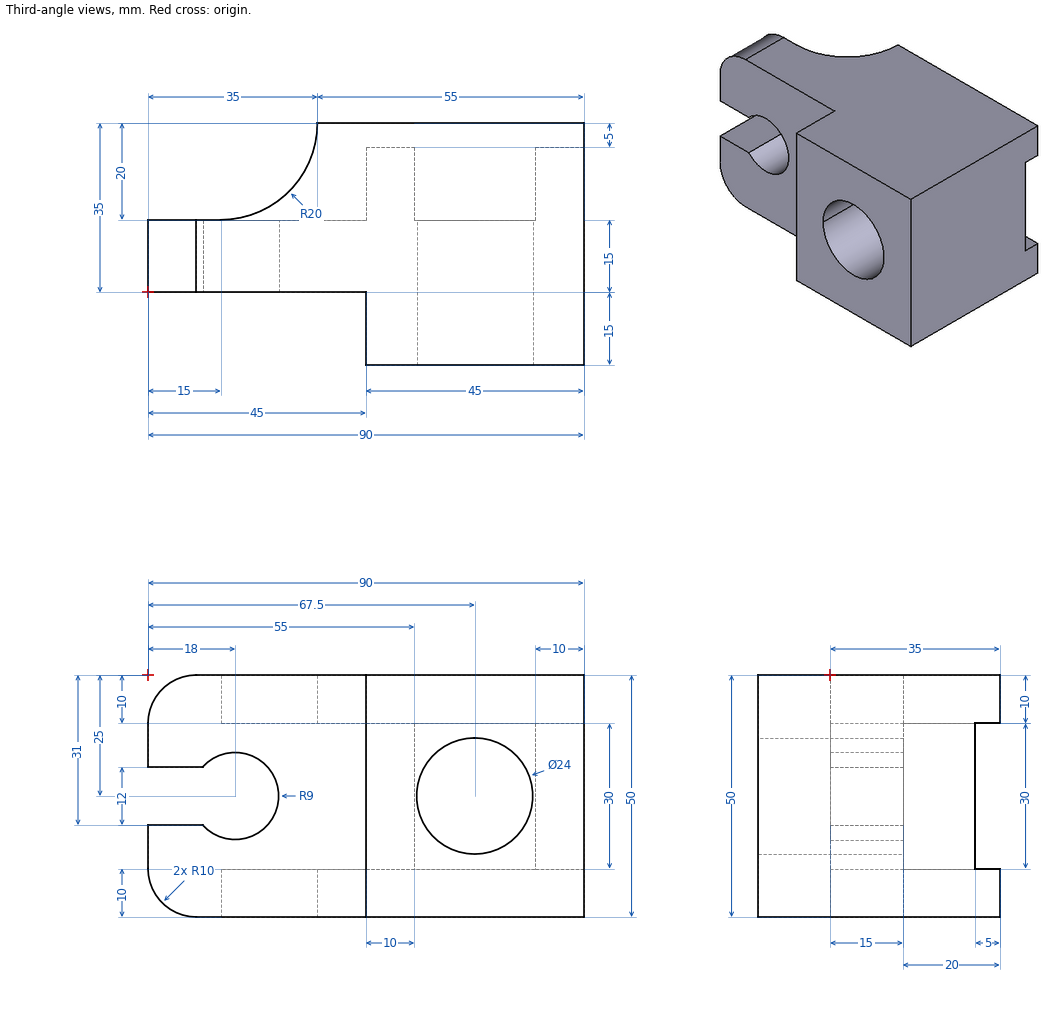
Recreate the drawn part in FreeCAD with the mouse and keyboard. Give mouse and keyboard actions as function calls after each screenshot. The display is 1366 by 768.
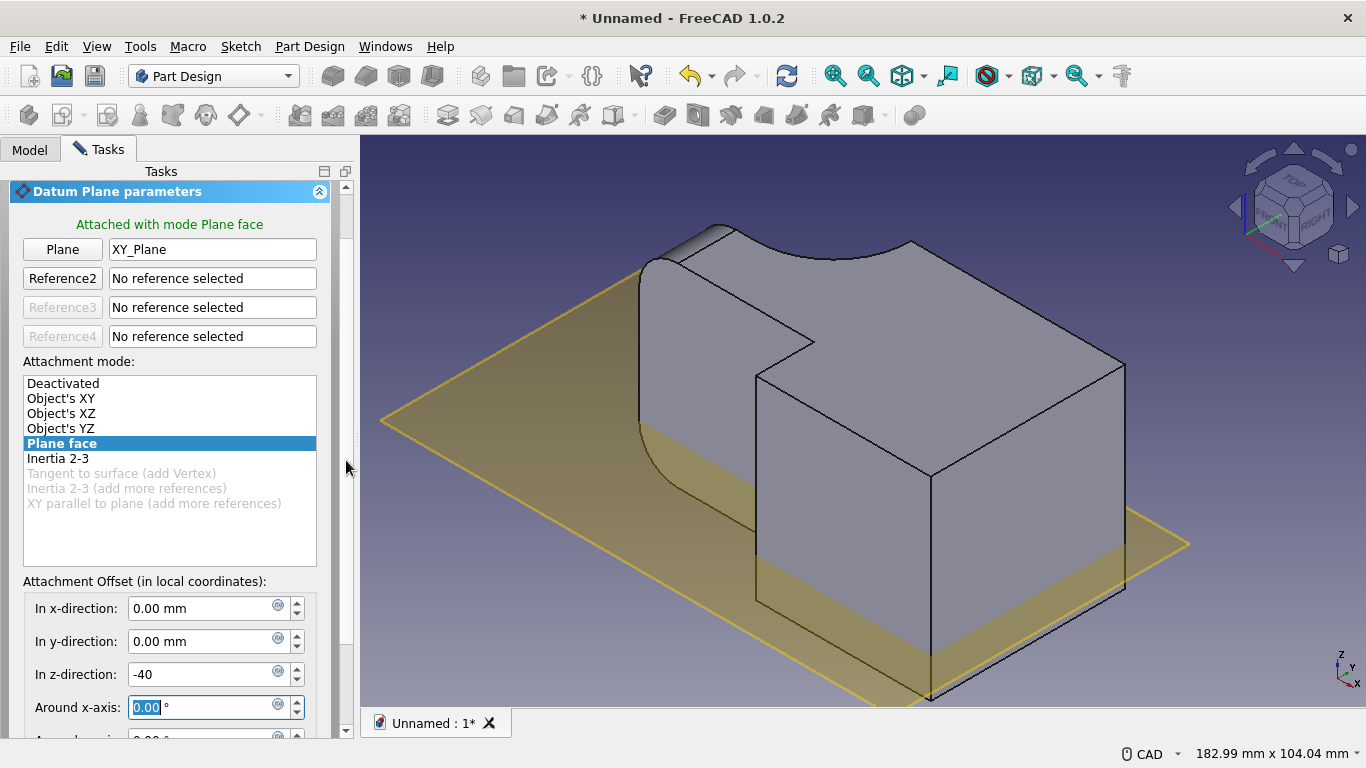
click(127, 210)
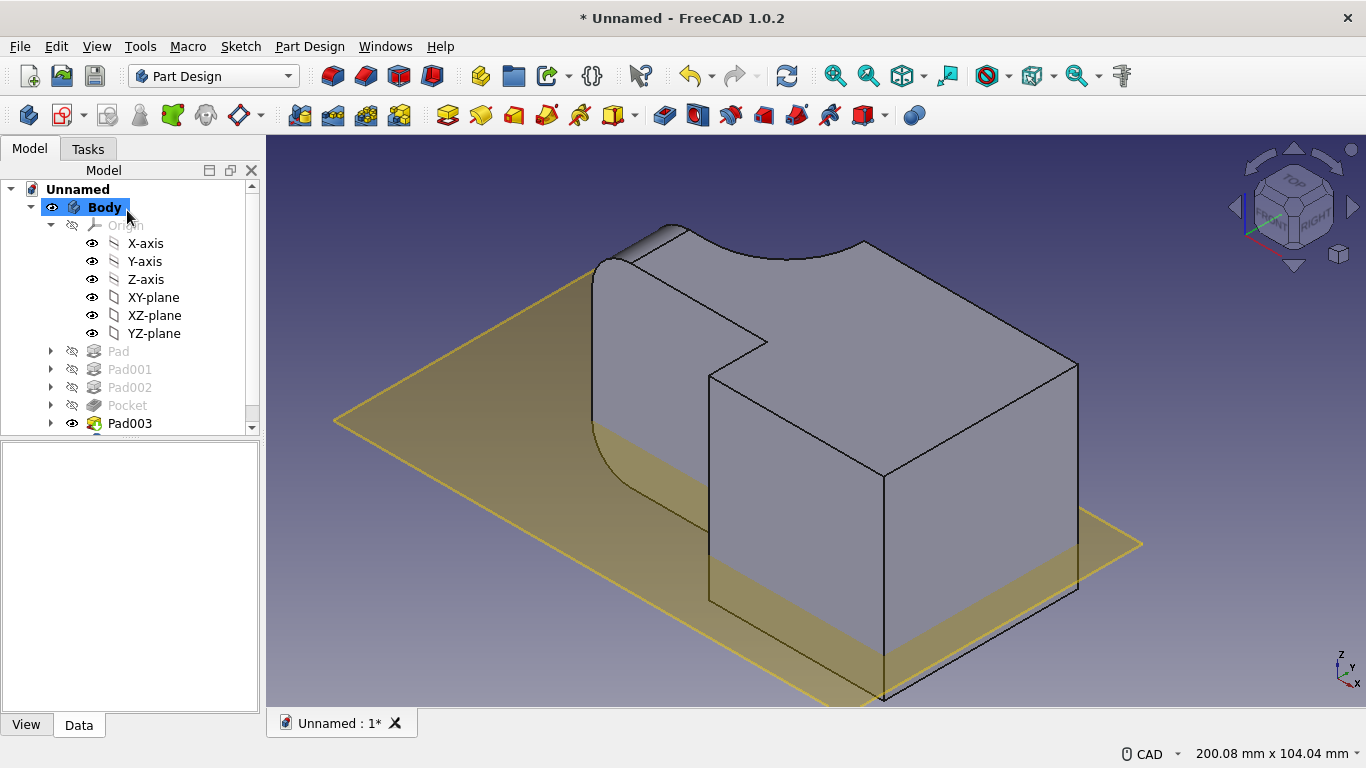
scroll(101, 311, down, 3)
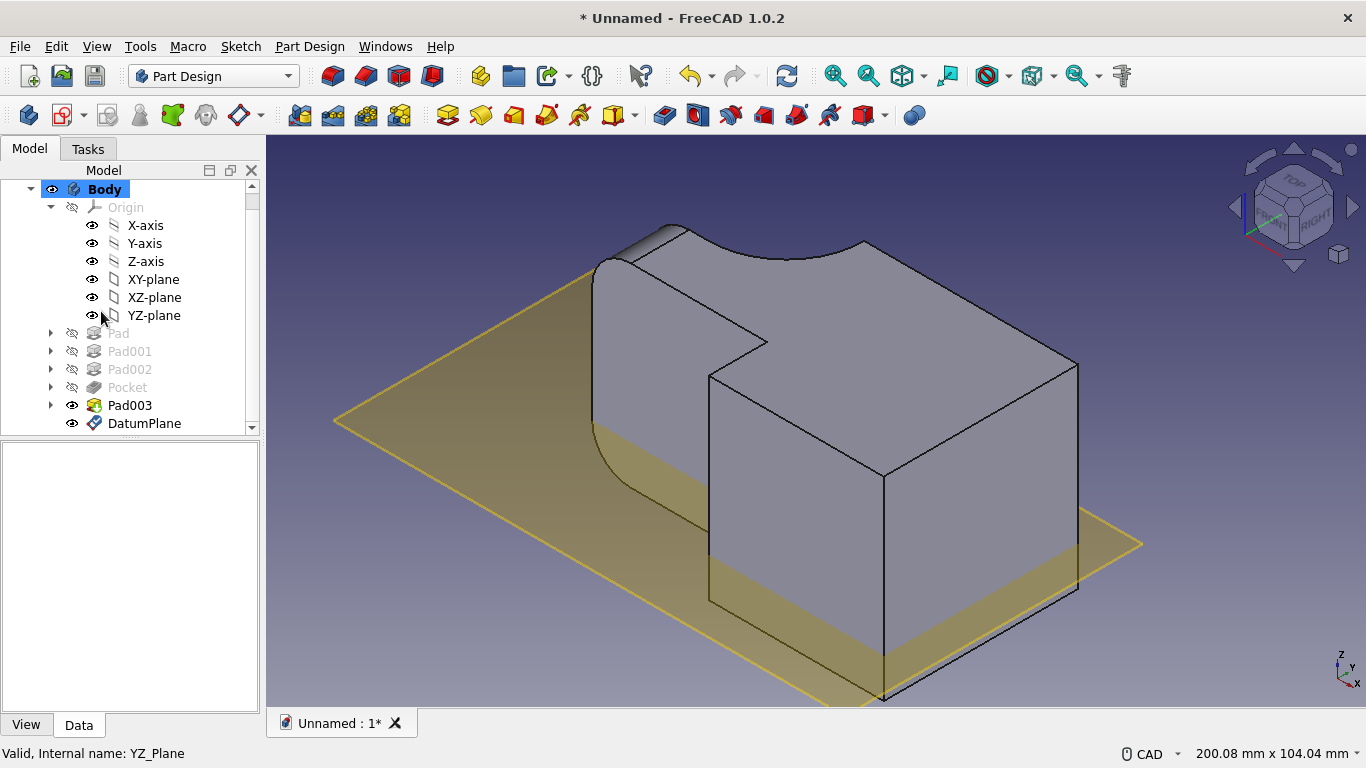
click(117, 423)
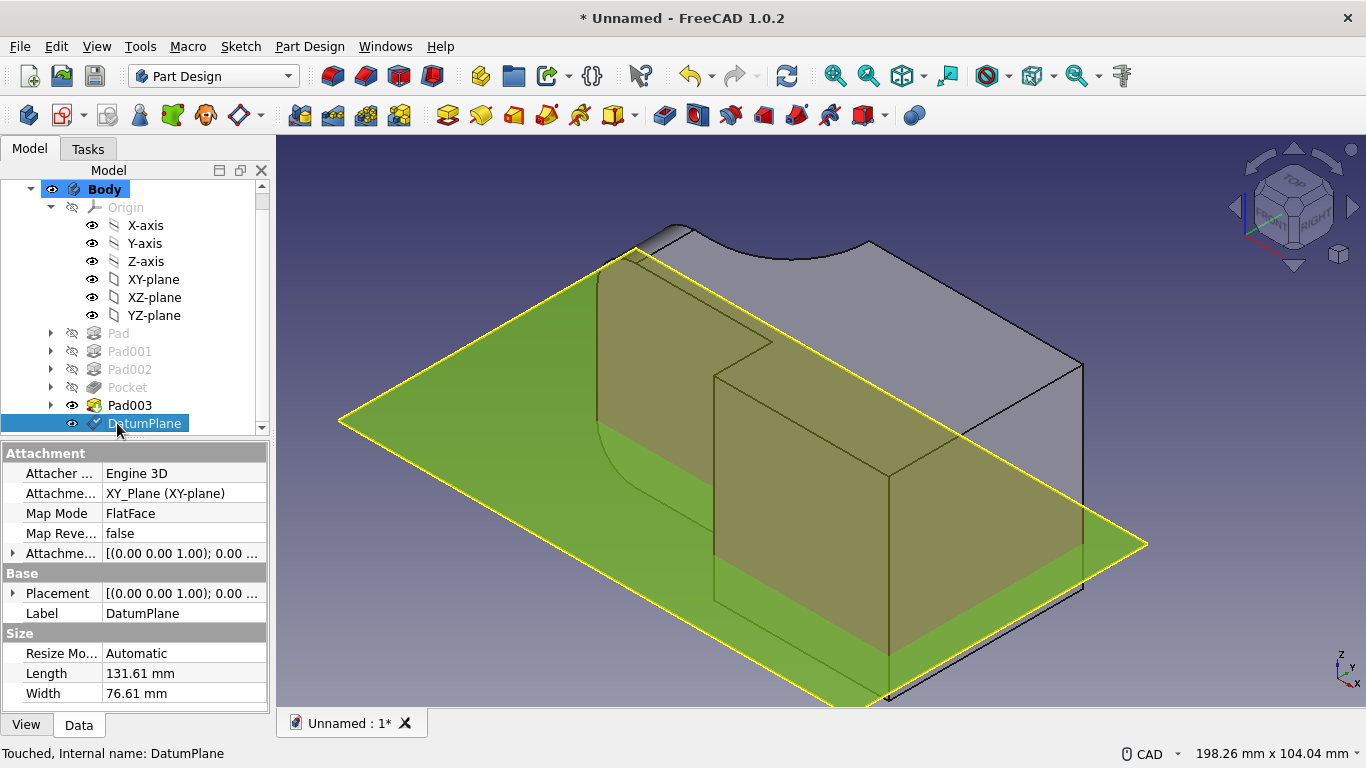
click(62, 116)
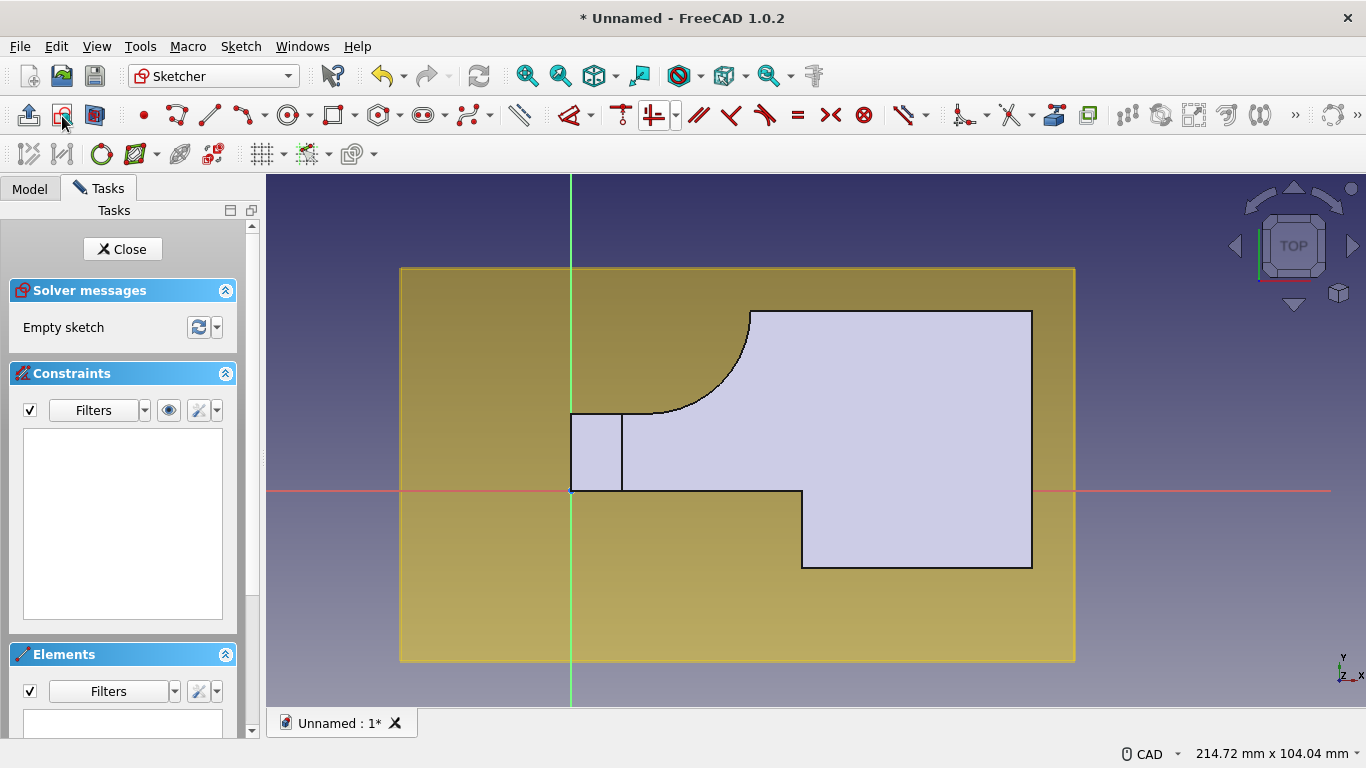
click(95, 116)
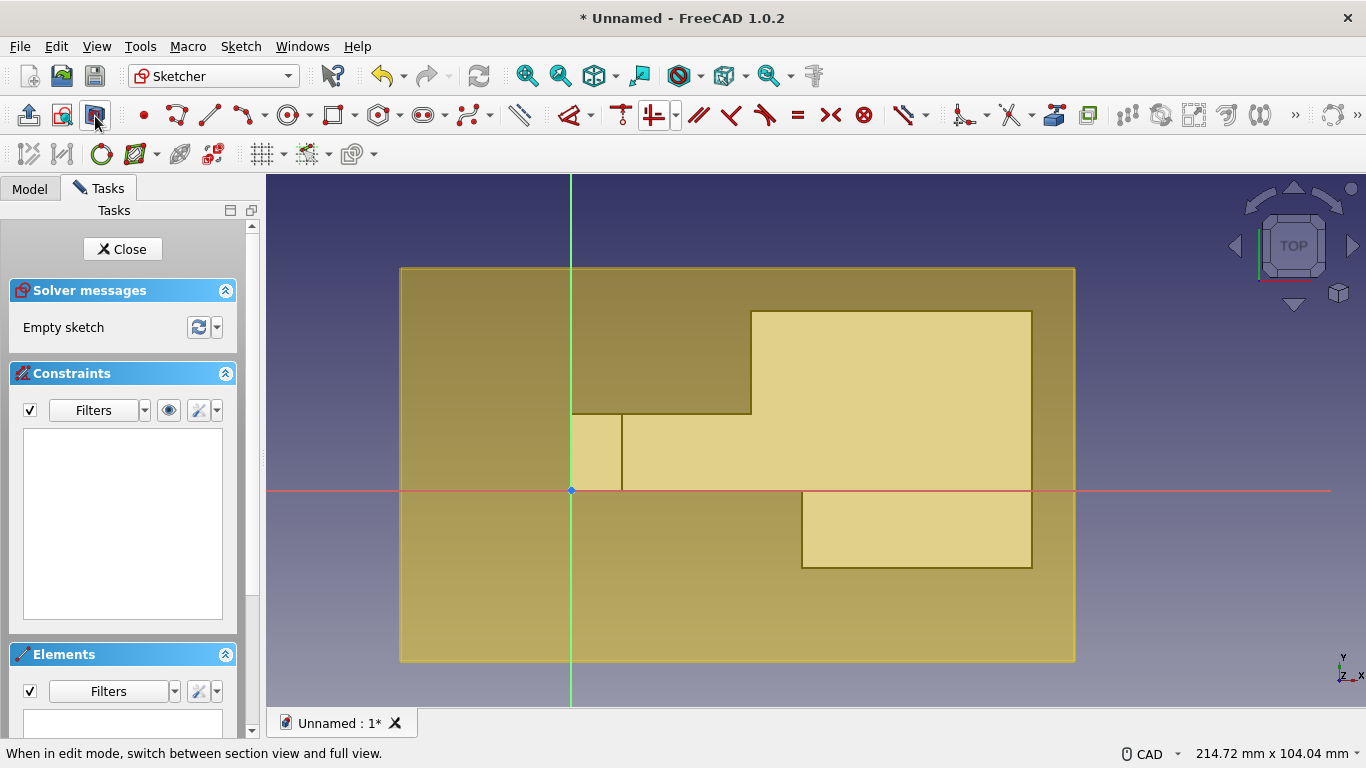
scroll(555, 353, up, 3)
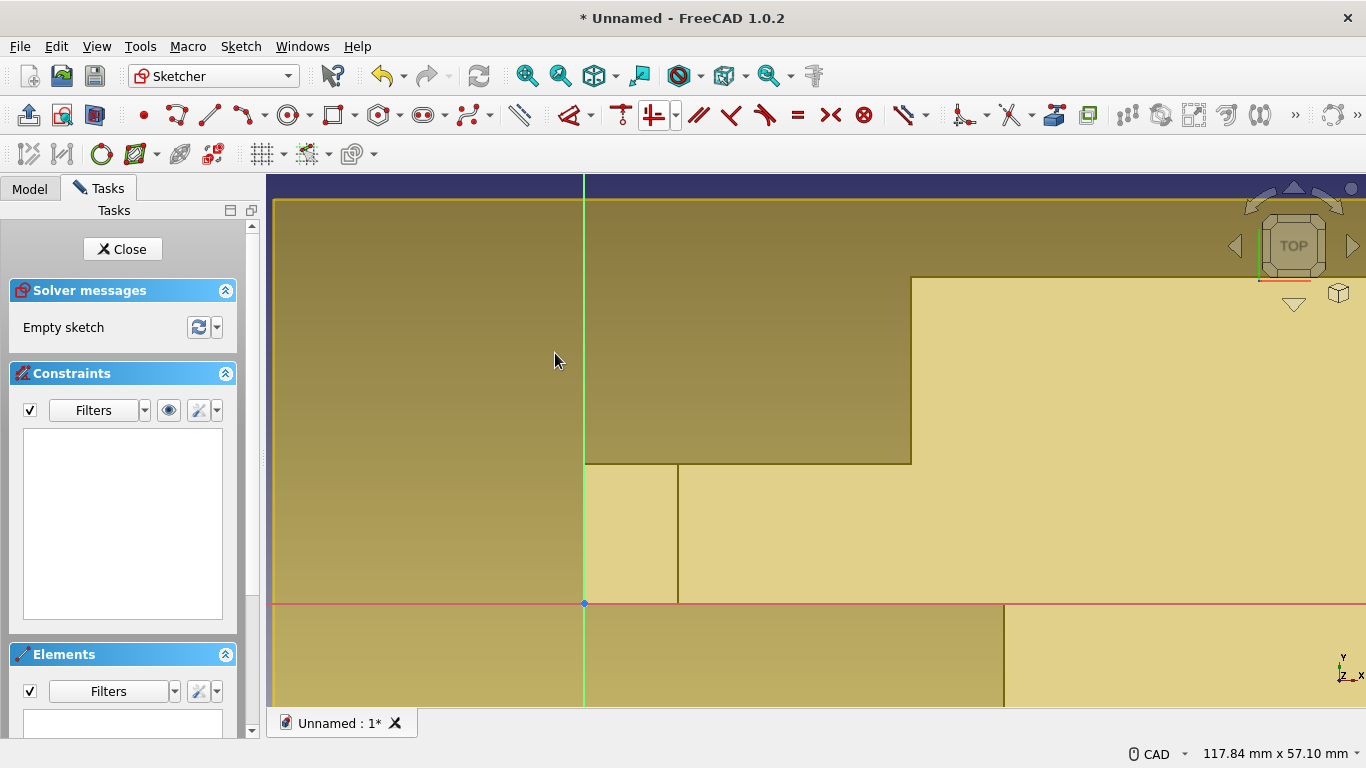
click(177, 116)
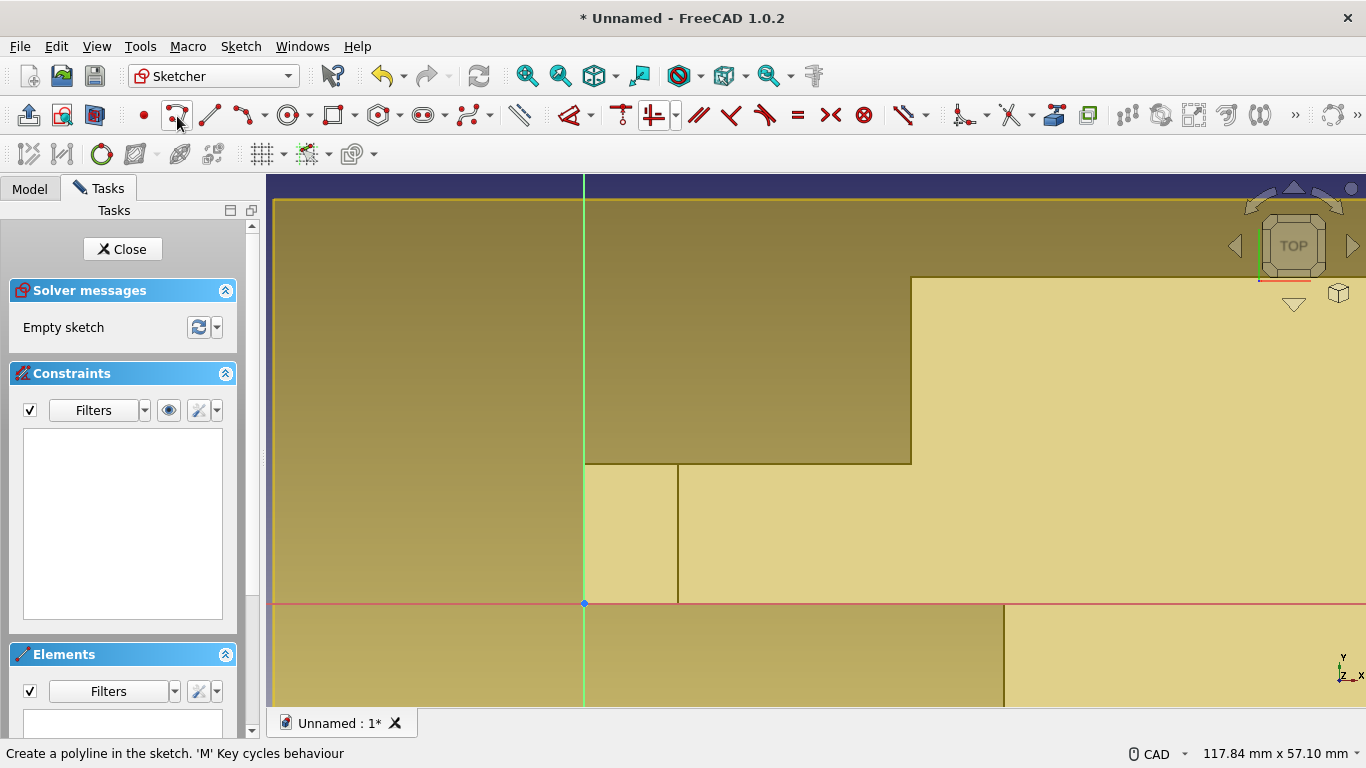
click(911, 277)
click(911, 464)
click(724, 464)
right_click(724, 464)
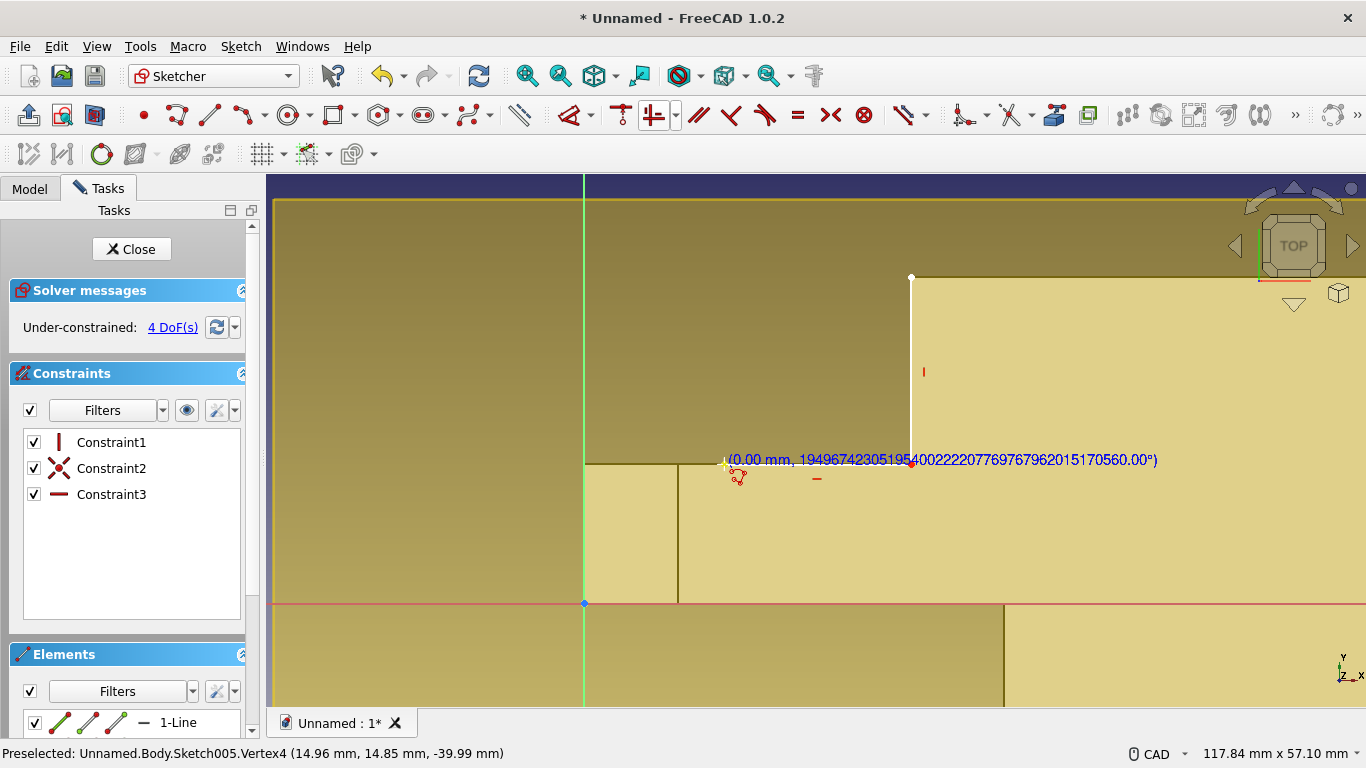
click(242, 116)